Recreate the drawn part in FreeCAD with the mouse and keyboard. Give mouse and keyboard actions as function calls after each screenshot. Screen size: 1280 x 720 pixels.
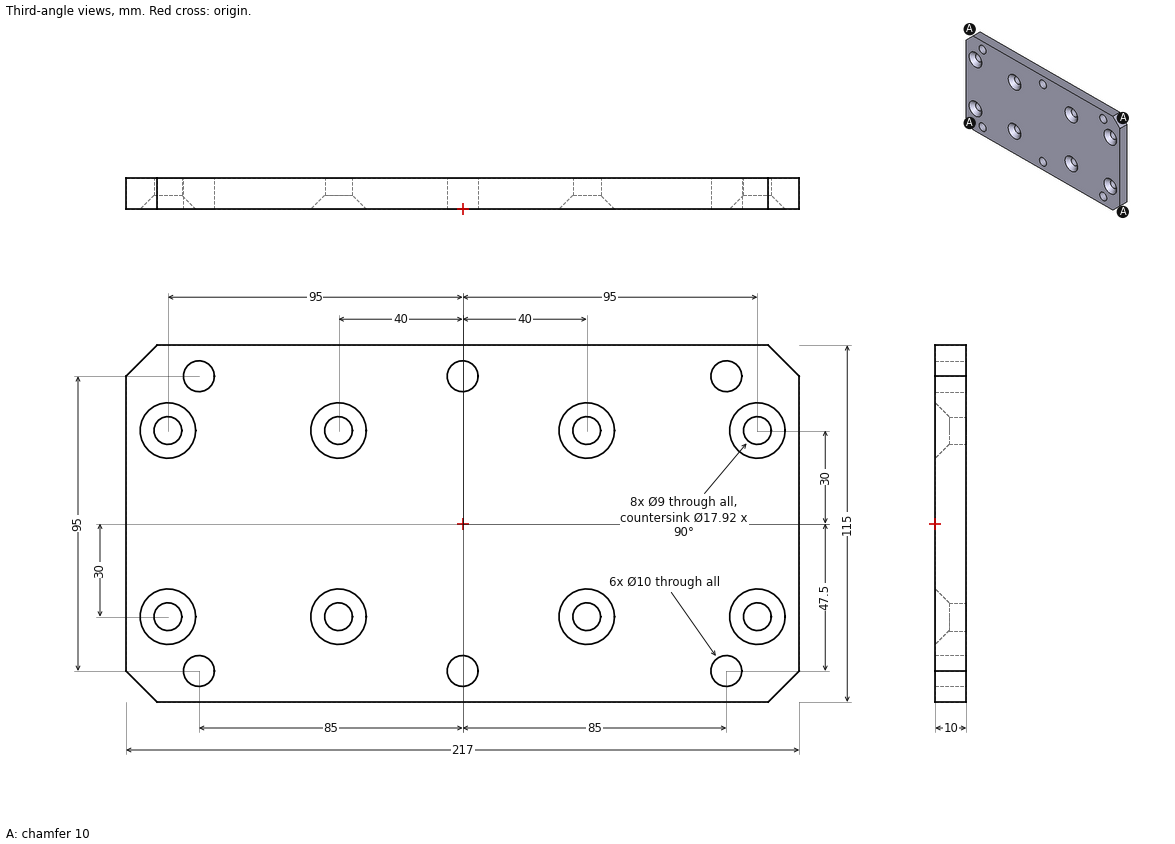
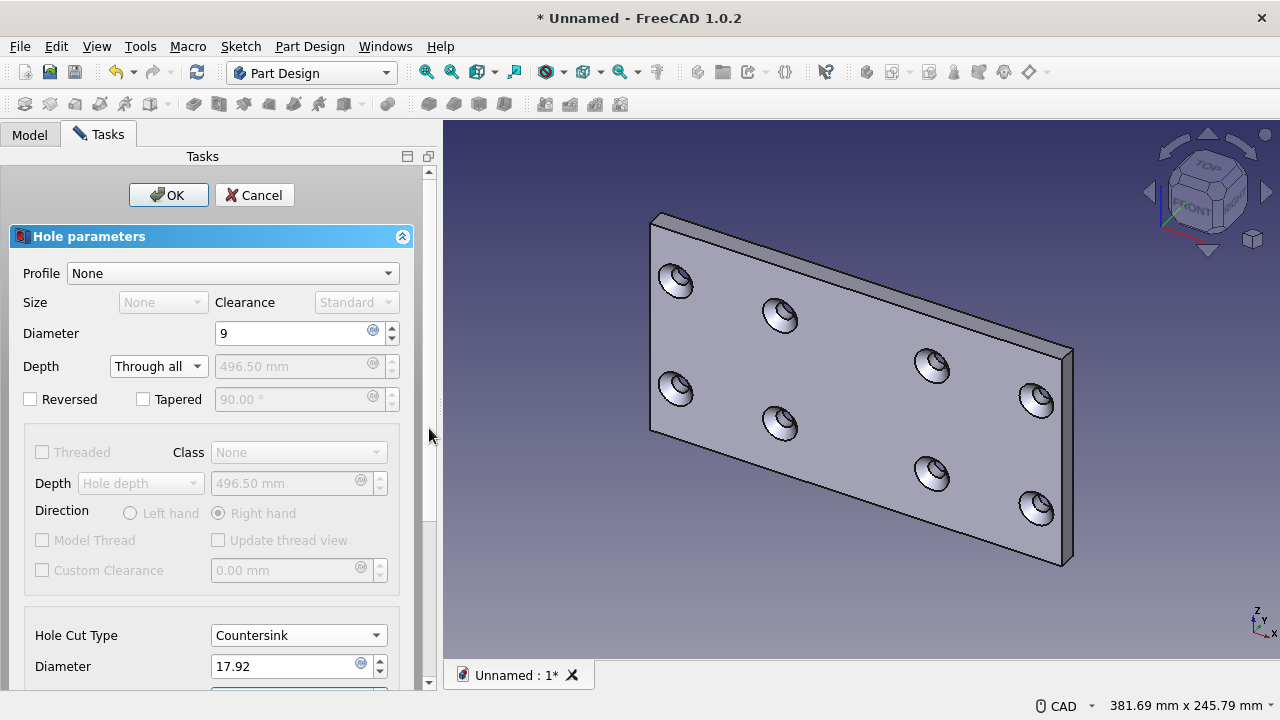
click(169, 195)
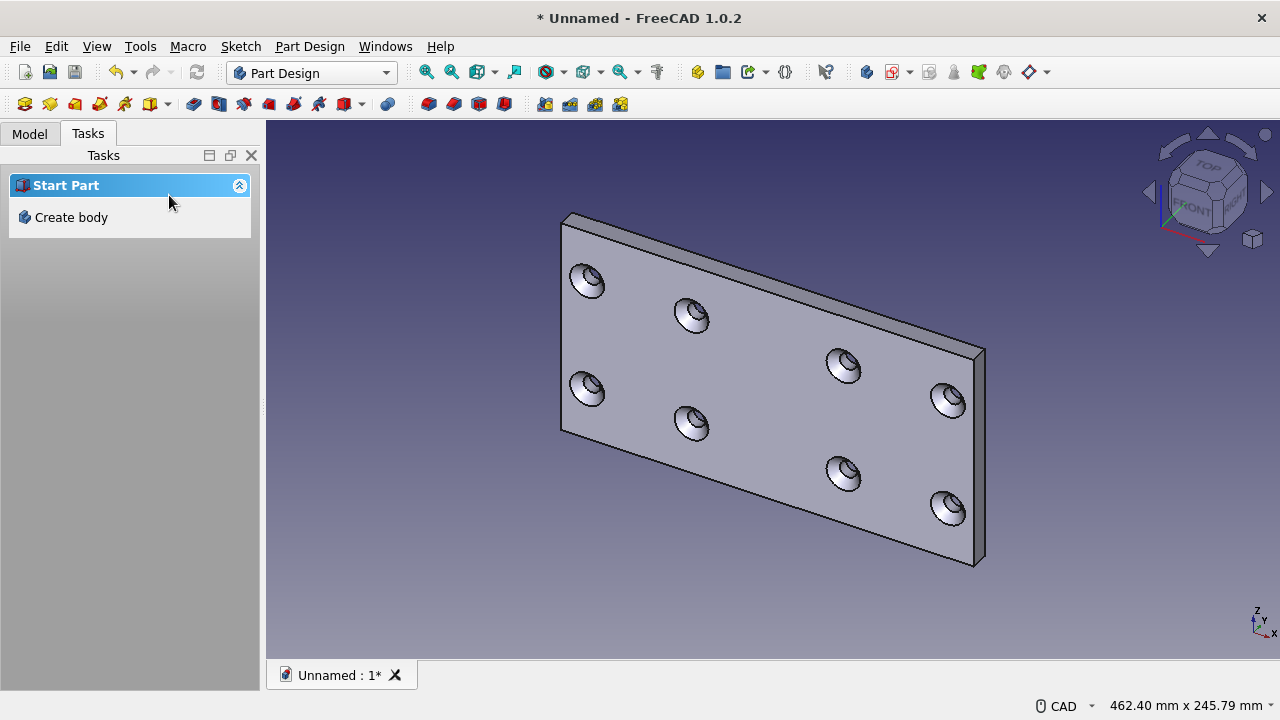
click(892, 72)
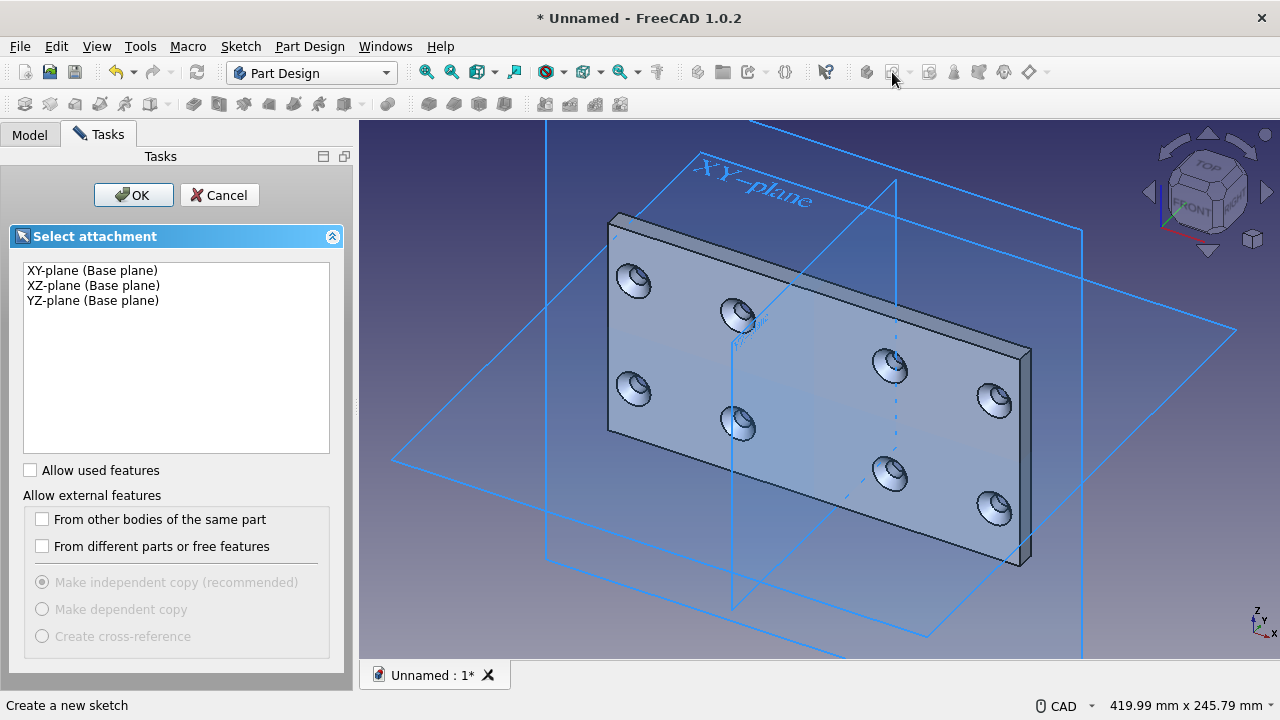
click(84, 286)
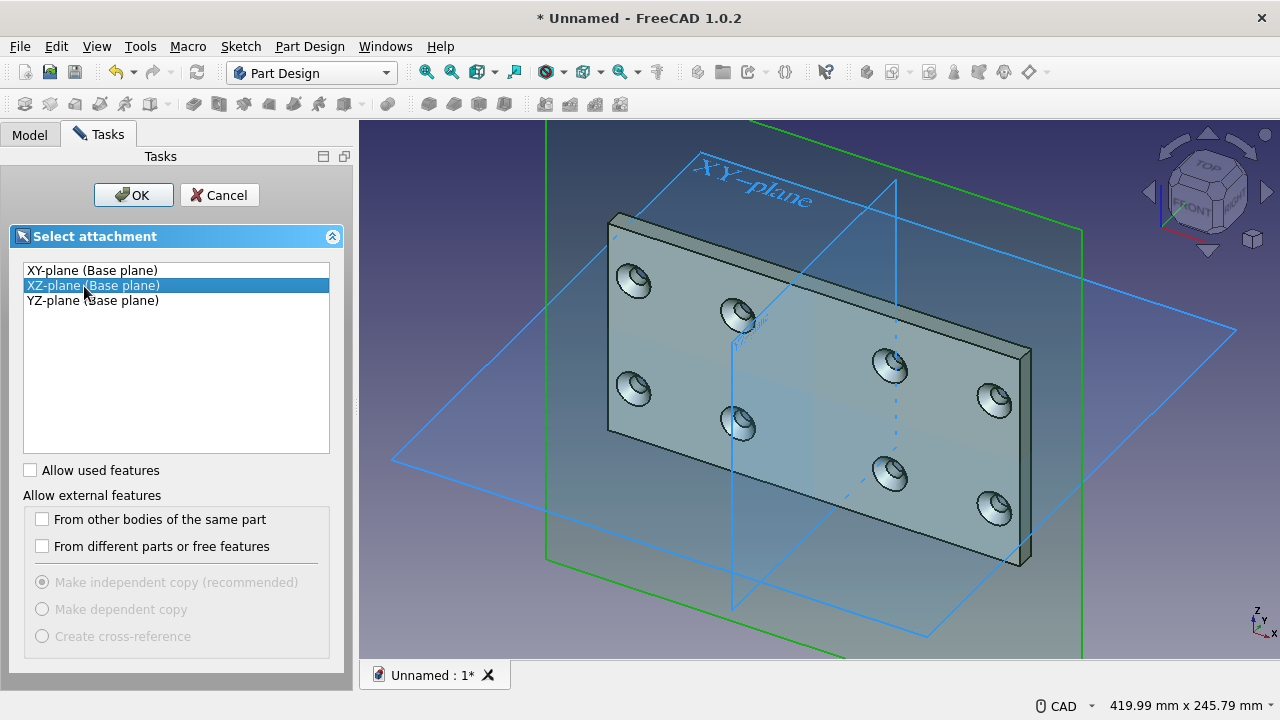
click(134, 195)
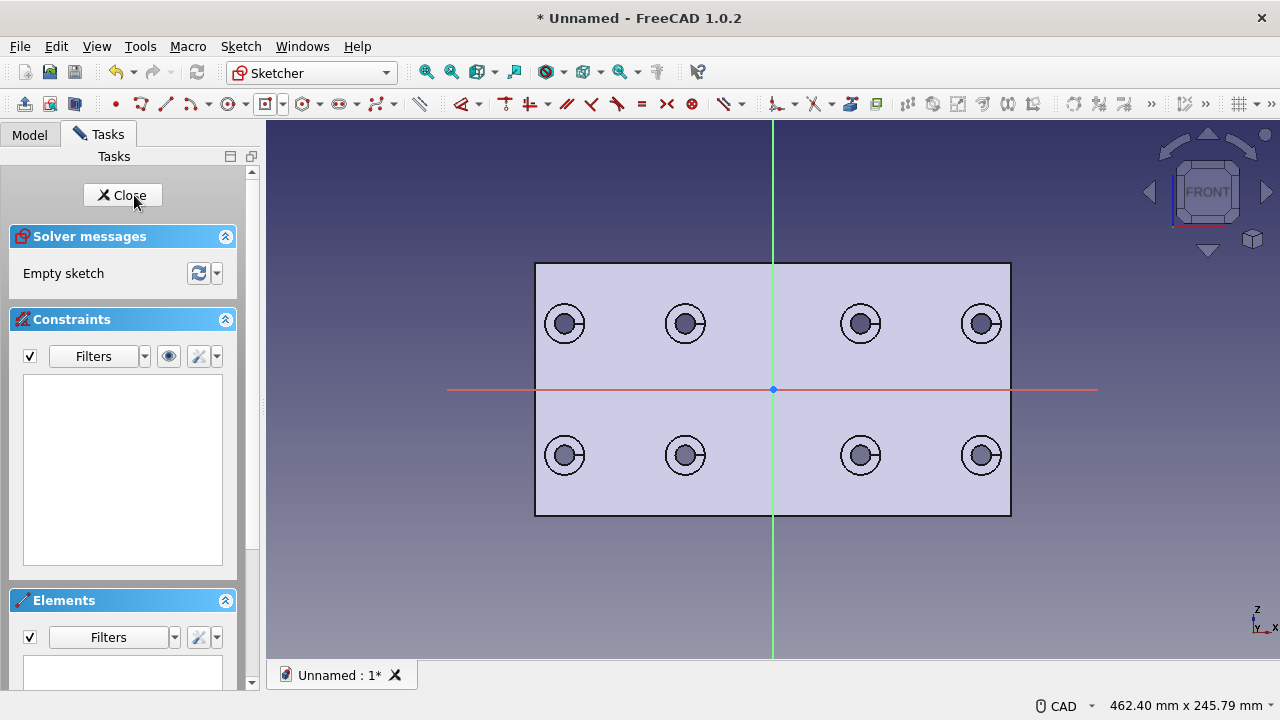
scroll(912, 390, up, 2)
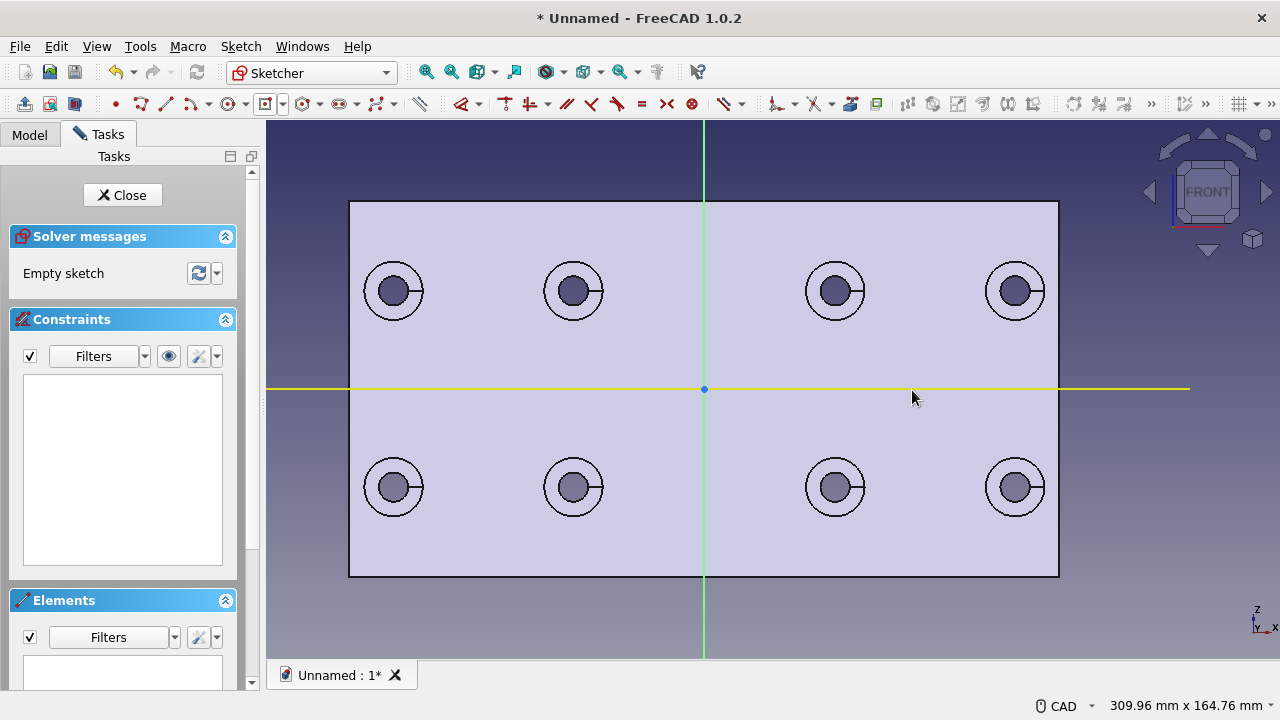
click(228, 104)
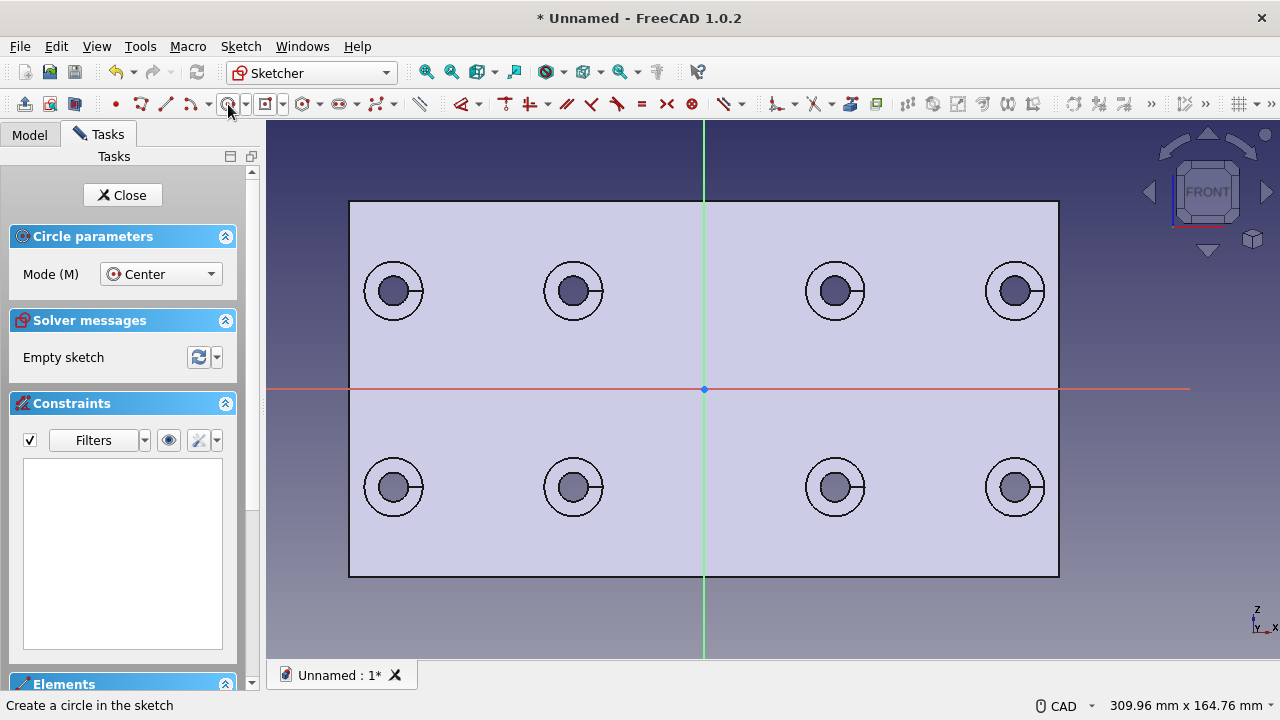
scroll(982, 544, up, 2)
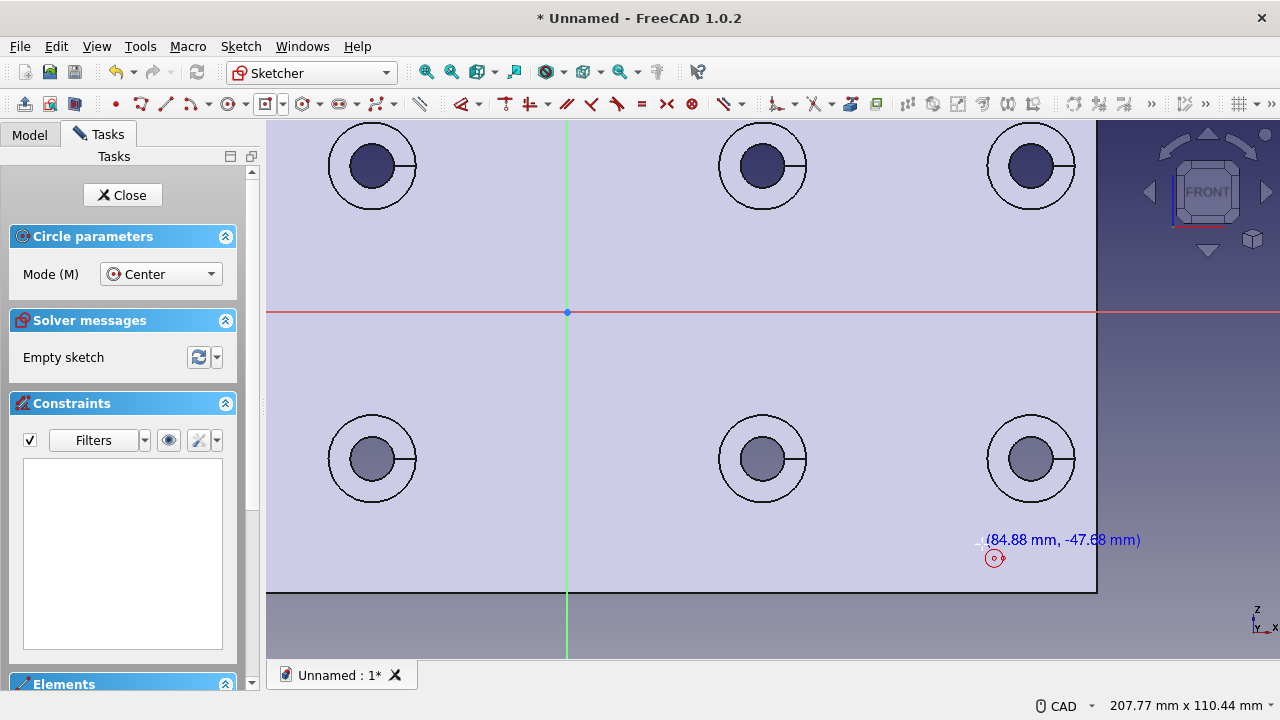
click(982, 544)
click(999, 527)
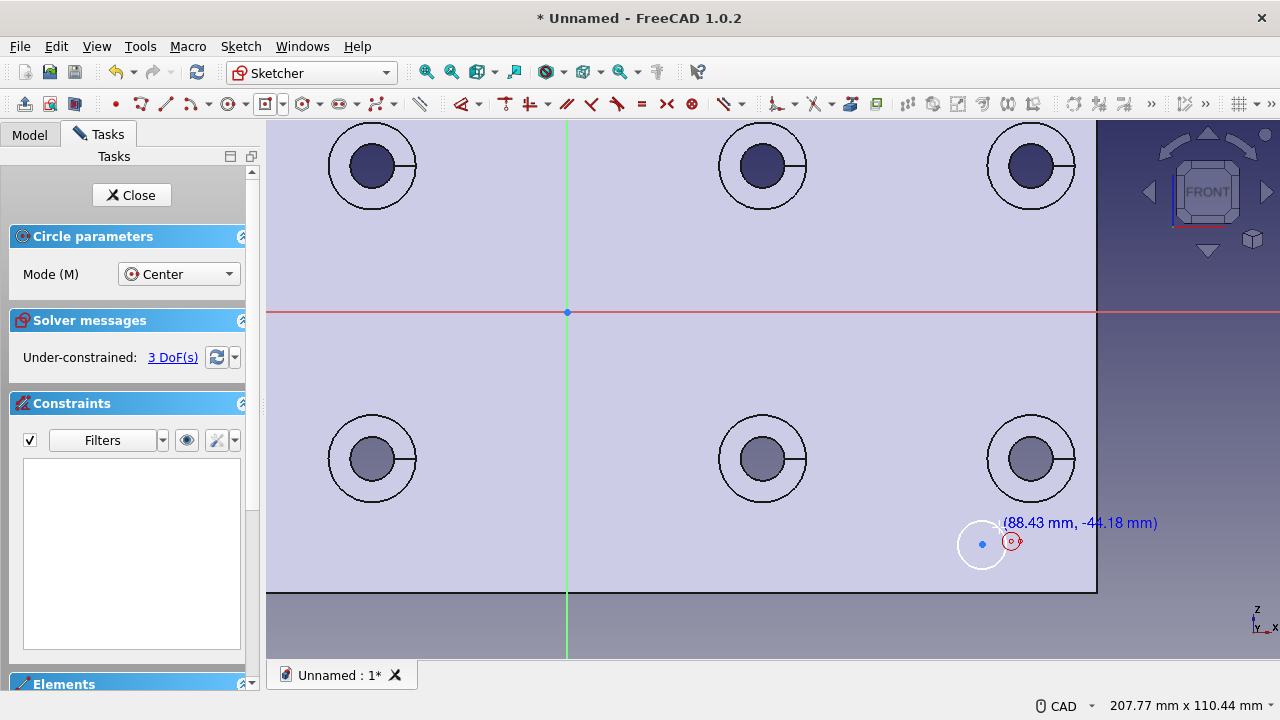
click(567, 544)
click(585, 527)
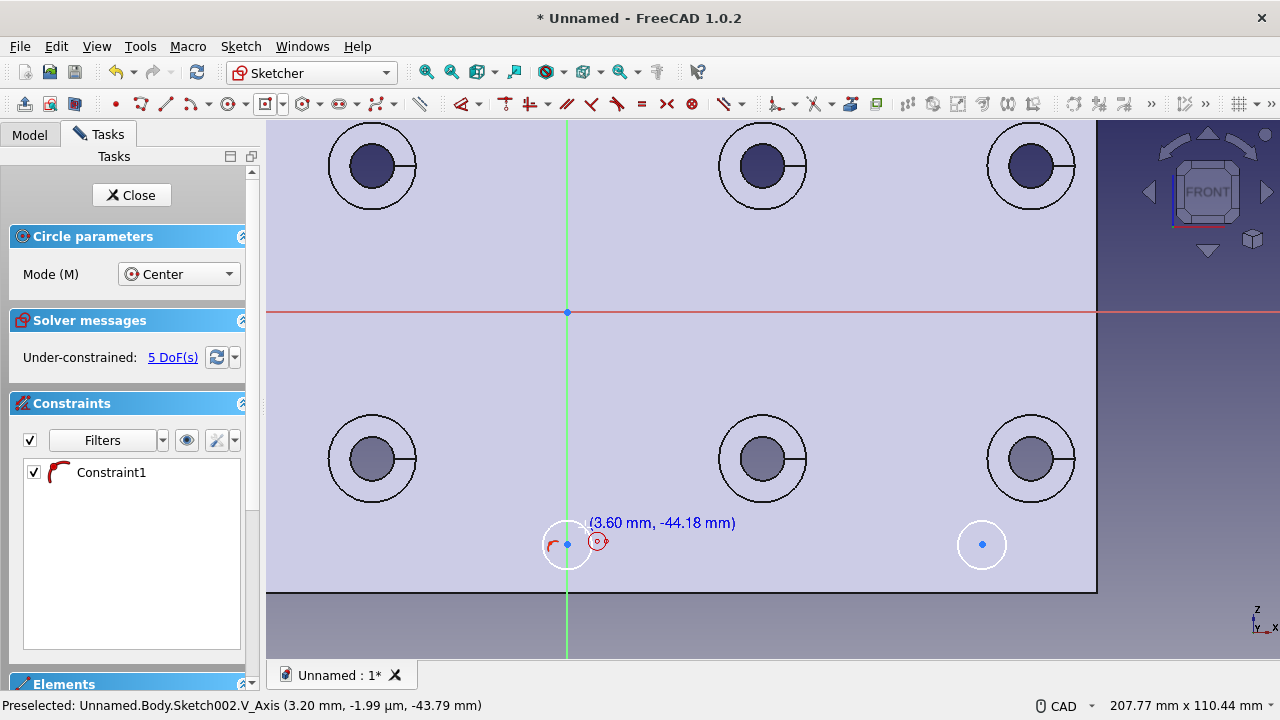
scroll(983, 546, down, 2)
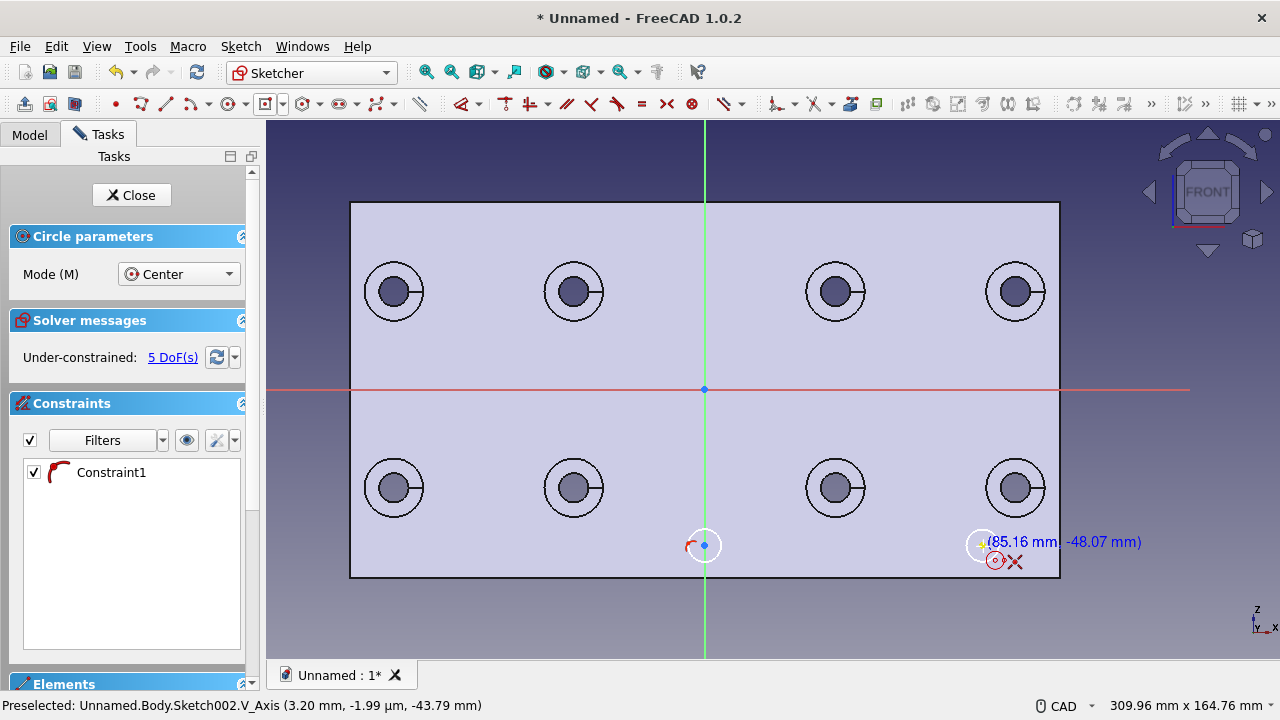
scroll(427, 545, up, 2)